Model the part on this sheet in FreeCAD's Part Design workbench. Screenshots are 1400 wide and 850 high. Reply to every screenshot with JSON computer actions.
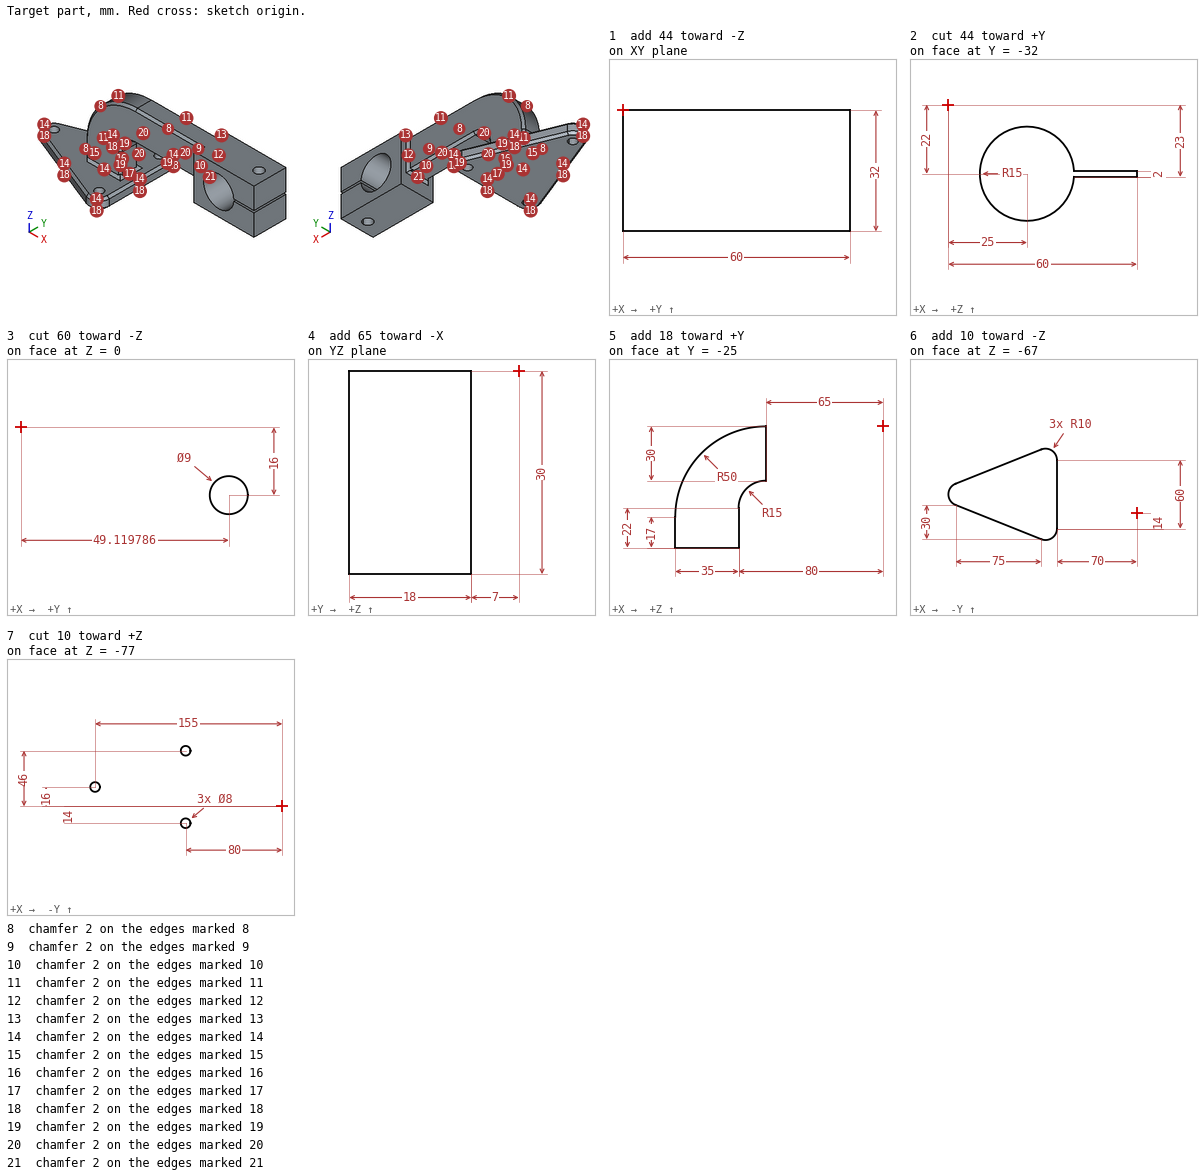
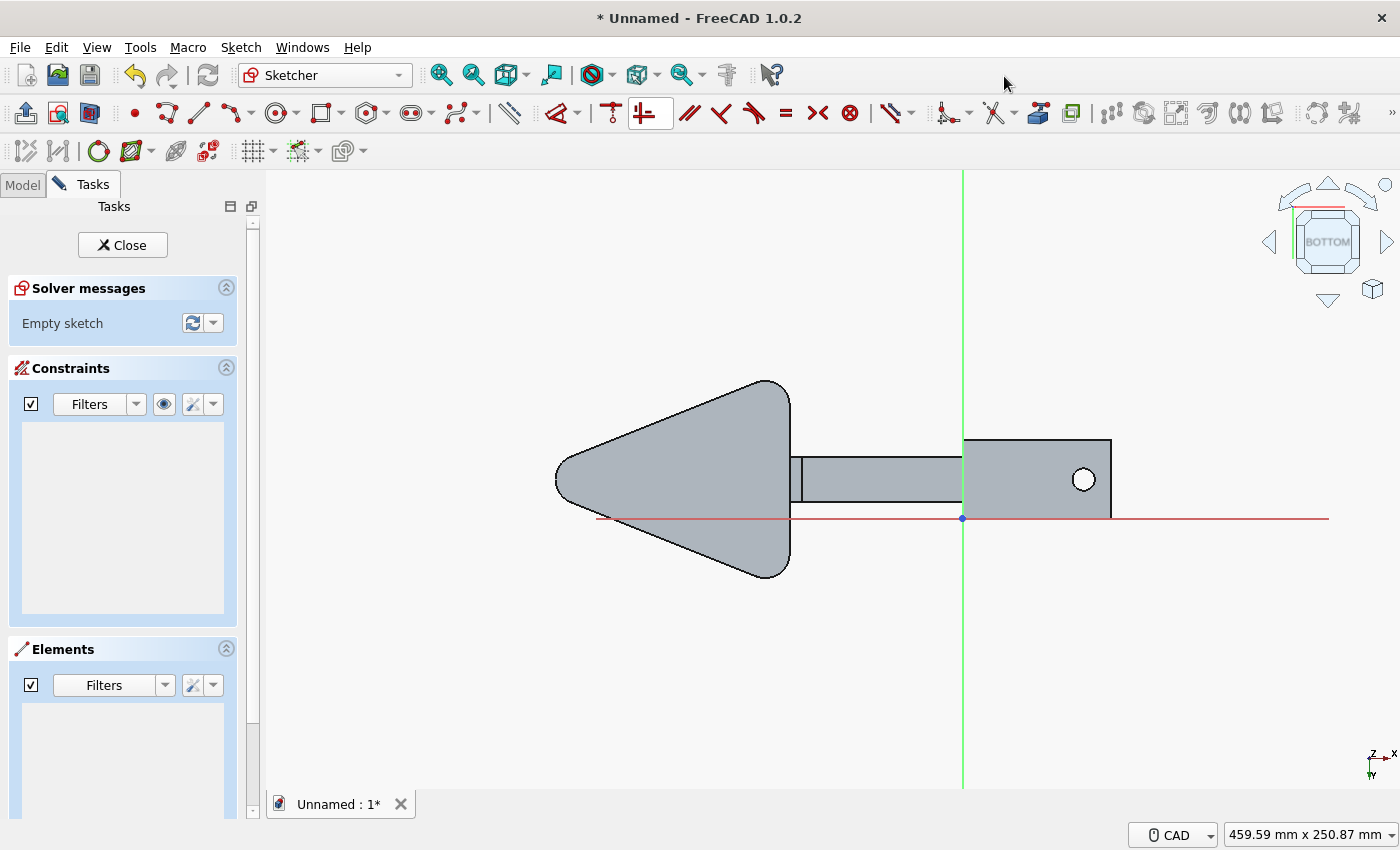
{"action": "scroll", "coordinate": [769, 479], "scroll_direction": "up", "scroll_amount": 3}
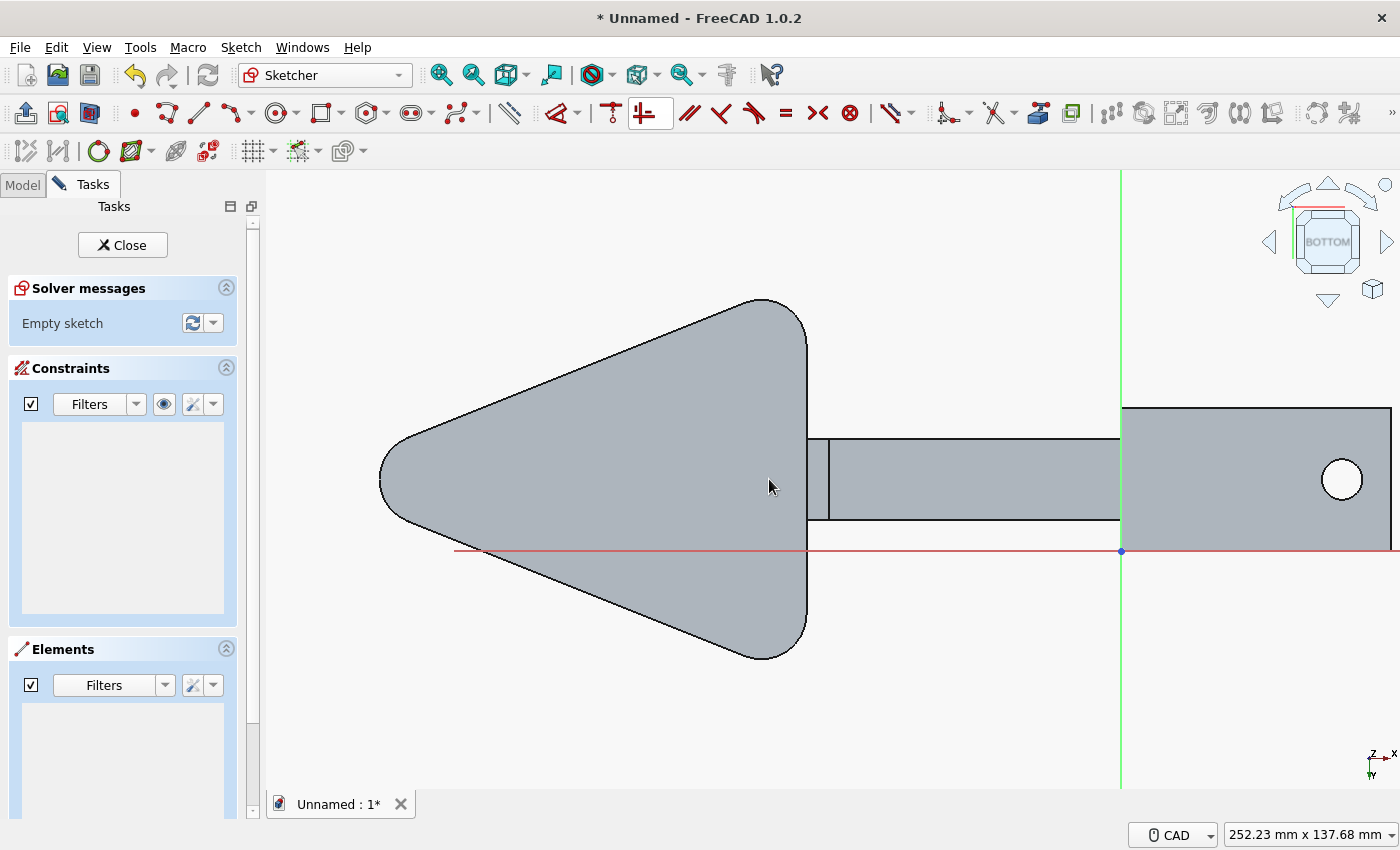
{"action": "left_click", "coordinate": [276, 114]}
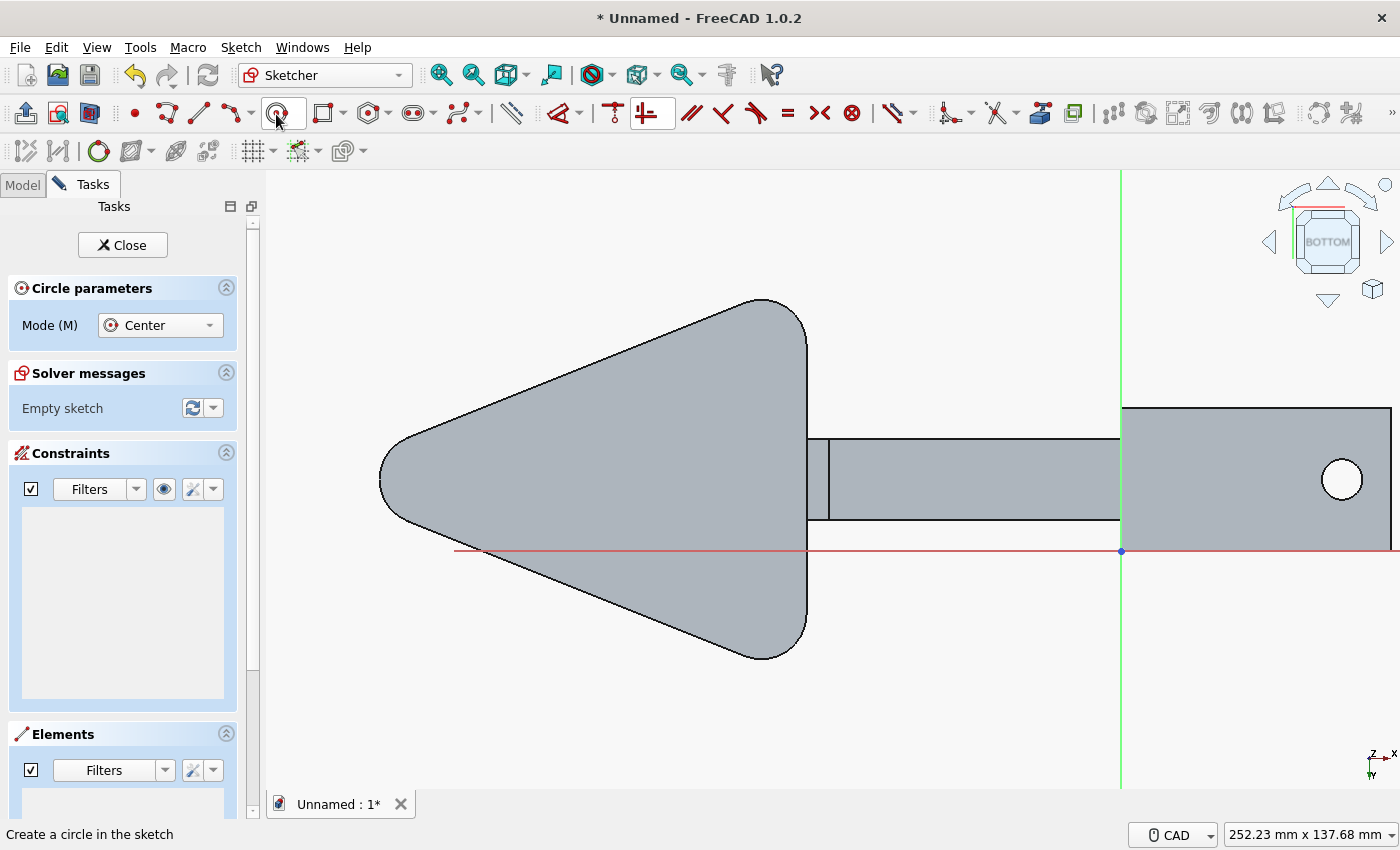
{"action": "scroll", "coordinate": [762, 614], "scroll_direction": "up", "scroll_amount": 2}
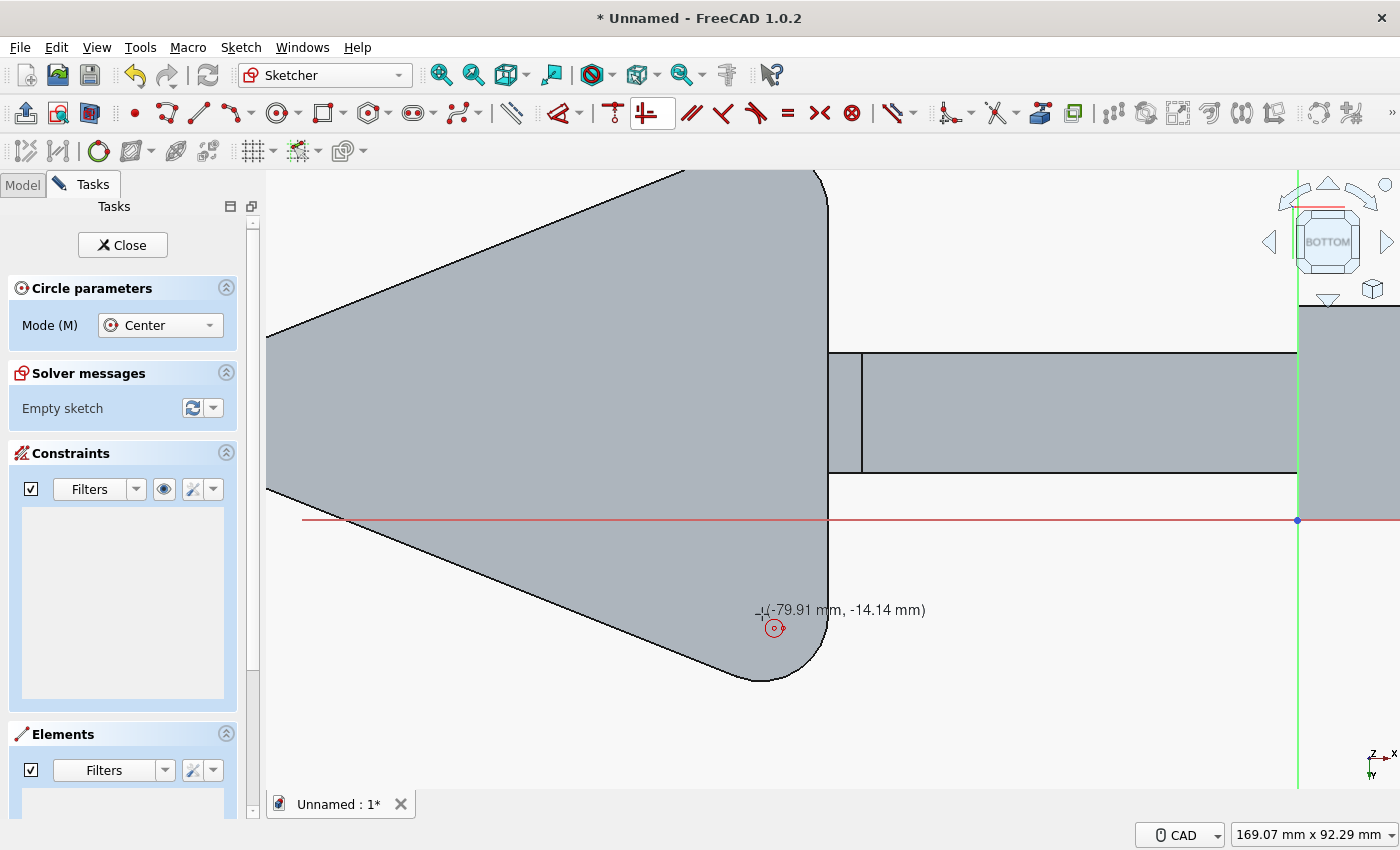
{"action": "left_click", "coordinate": [761, 614]}
{"action": "mouse_move", "coordinate": [780, 595]}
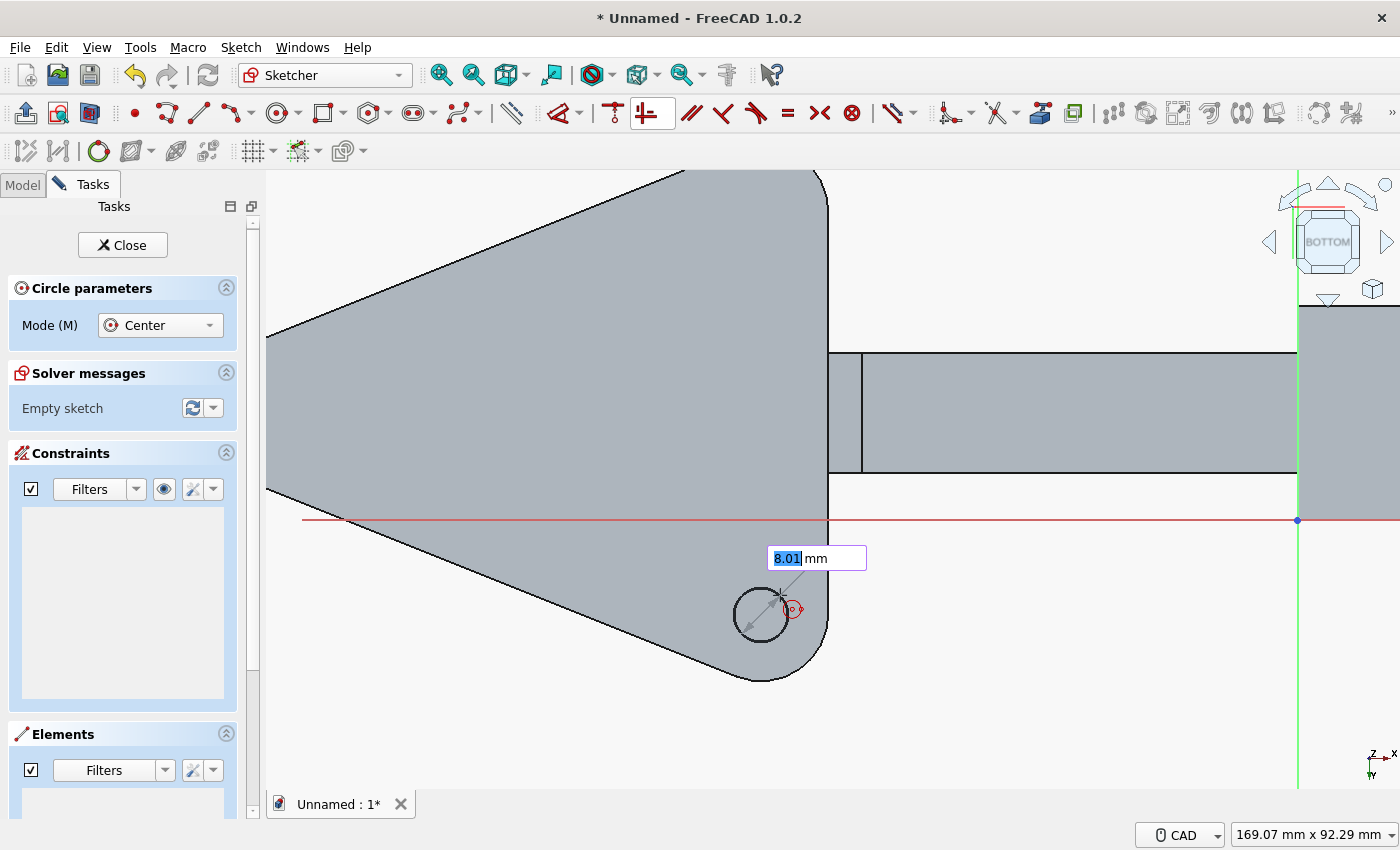
{"action": "type", "text": "8"}
{"action": "key", "text": "Return"}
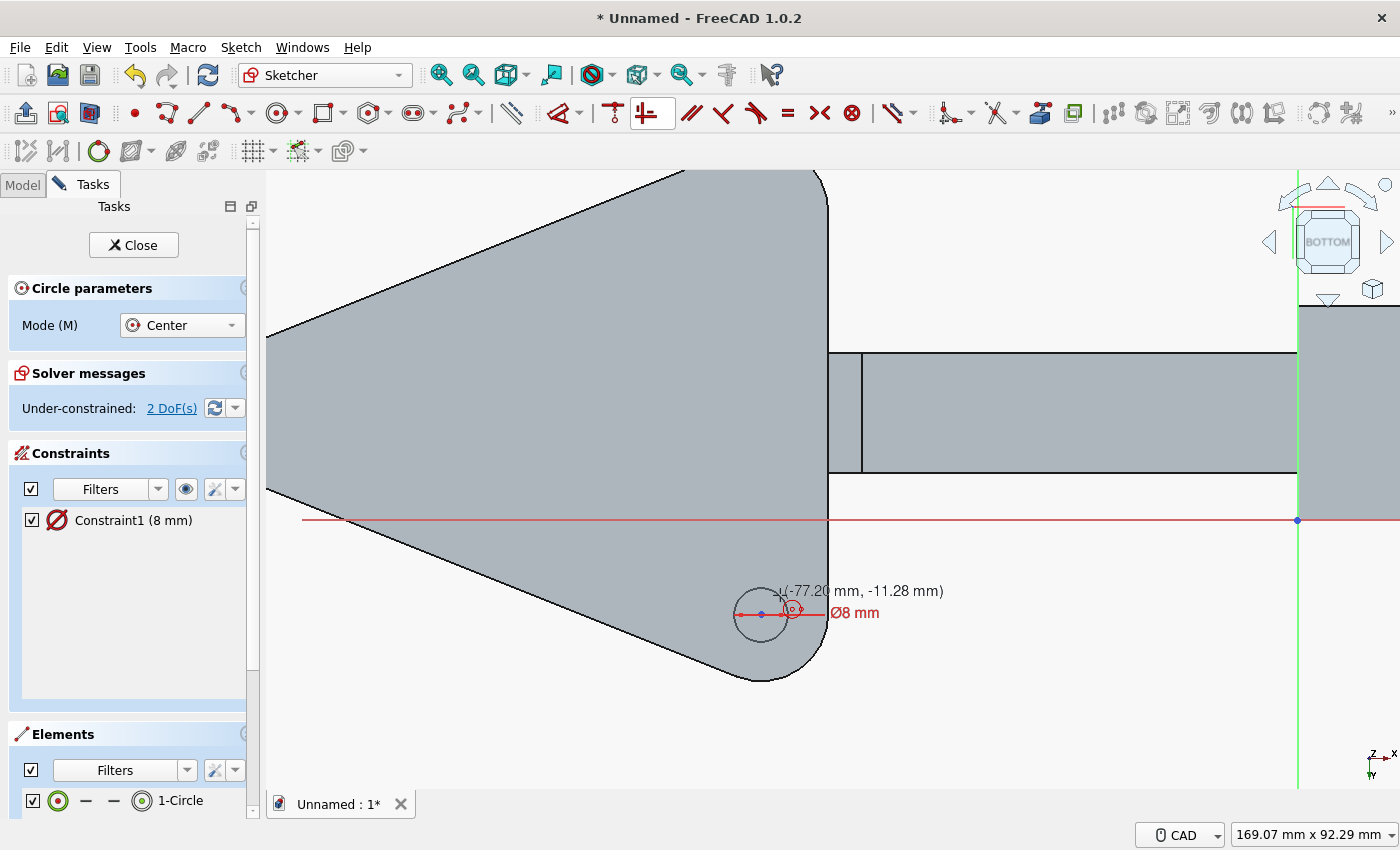
{"action": "scroll", "coordinate": [764, 615], "scroll_direction": "down", "scroll_amount": 2}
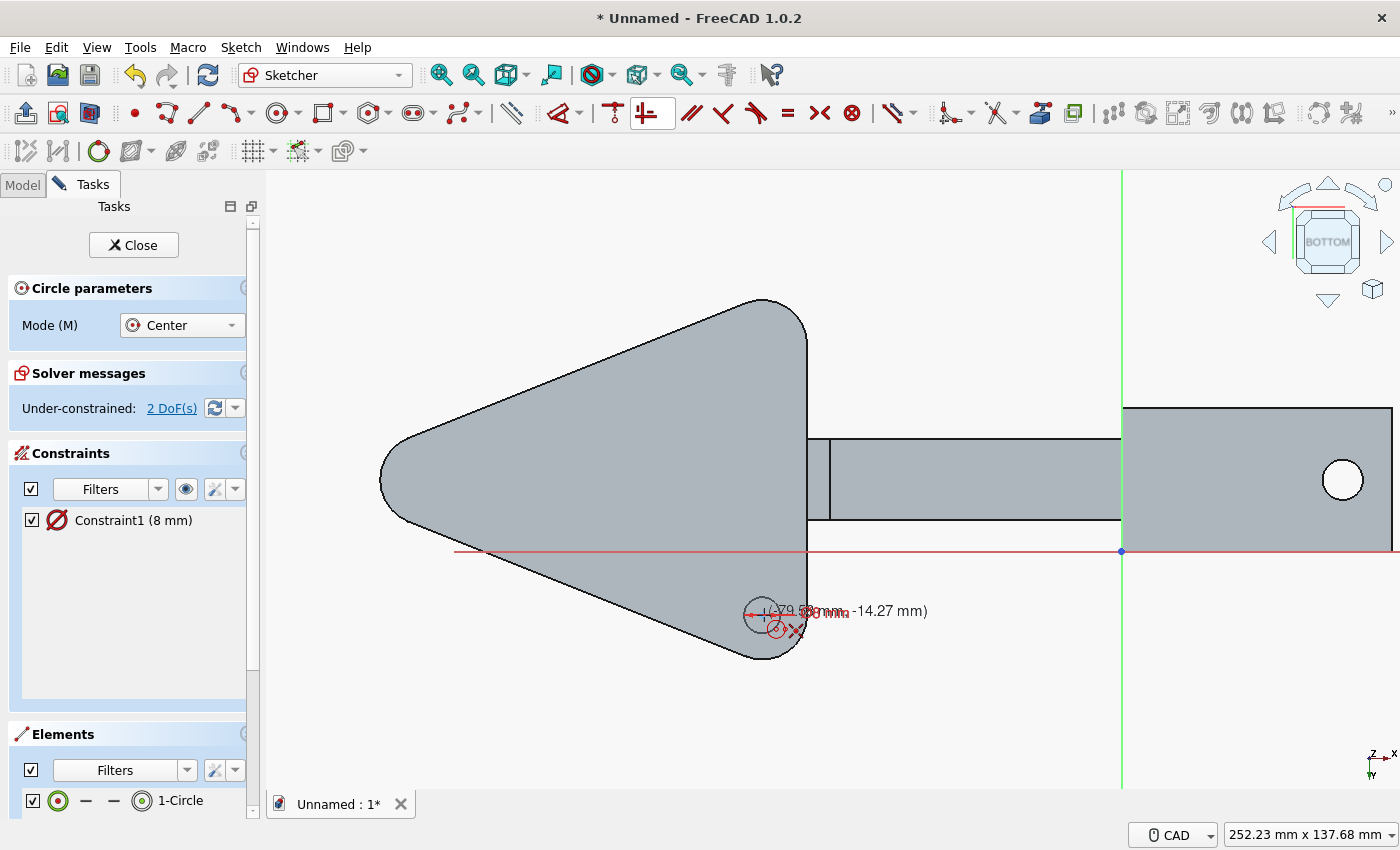
{"action": "scroll", "coordinate": [425, 480], "scroll_direction": "up", "scroll_amount": 2}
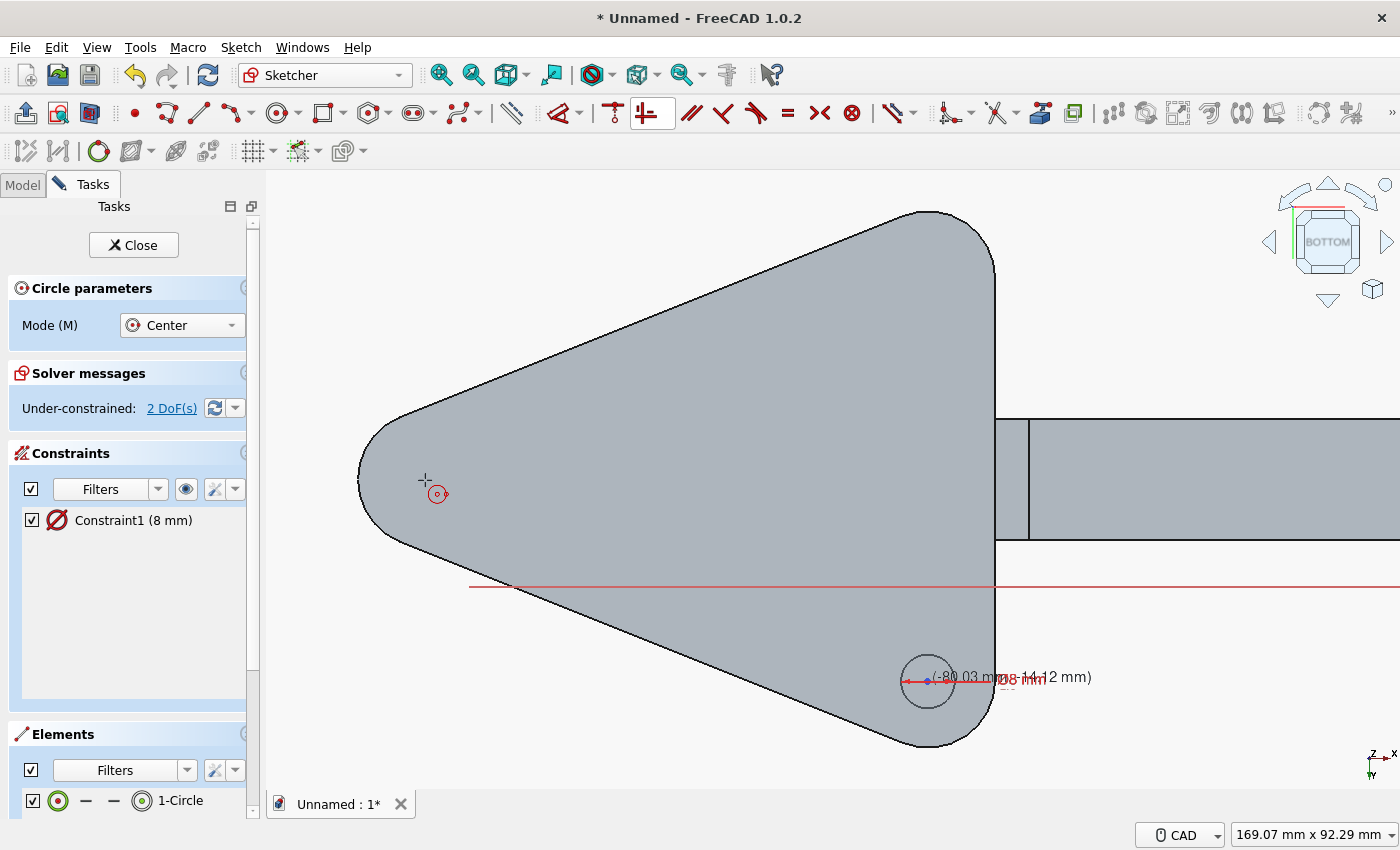
{"action": "left_click", "coordinate": [425, 480]}
{"action": "mouse_move", "coordinate": [444, 461]}